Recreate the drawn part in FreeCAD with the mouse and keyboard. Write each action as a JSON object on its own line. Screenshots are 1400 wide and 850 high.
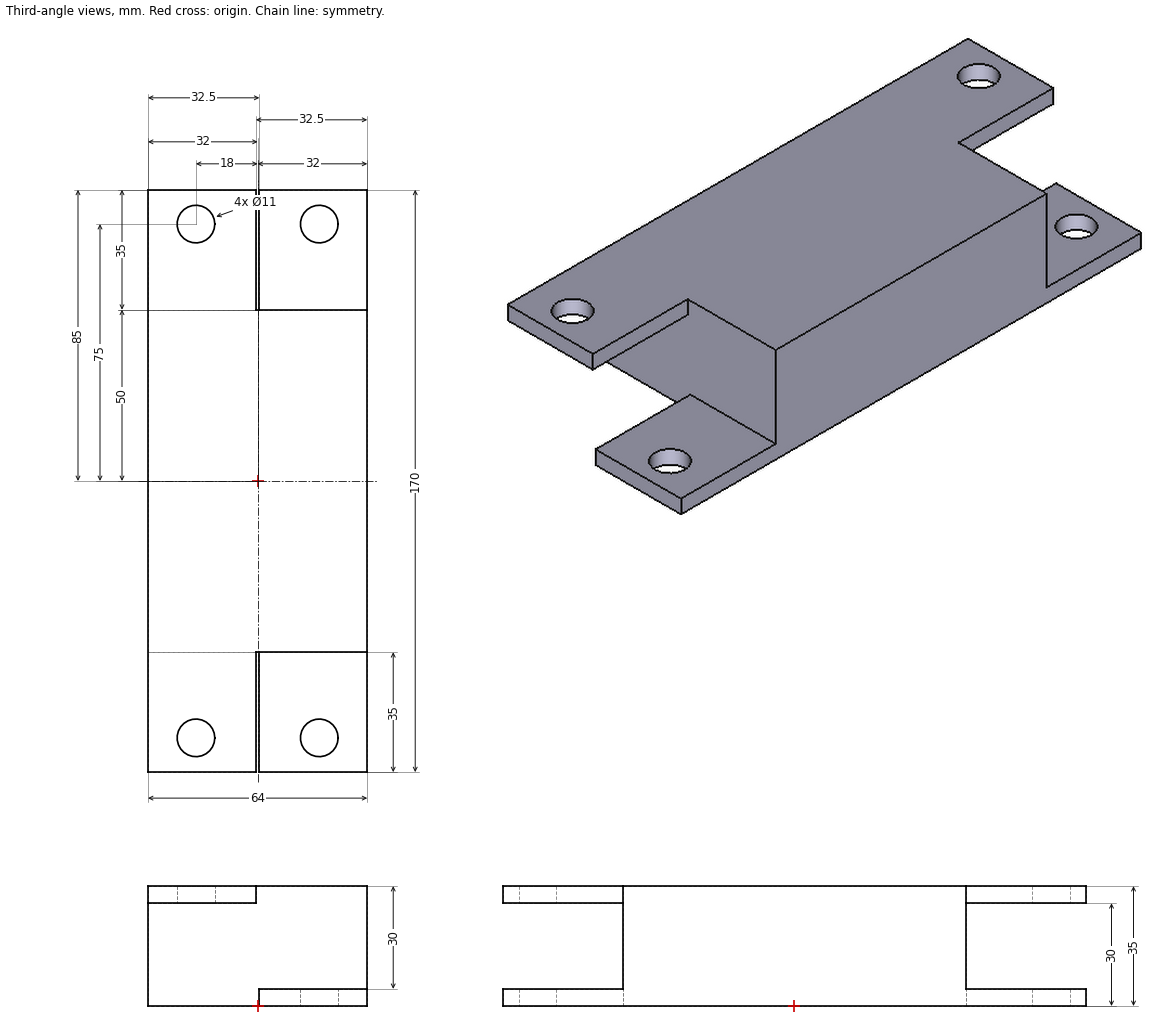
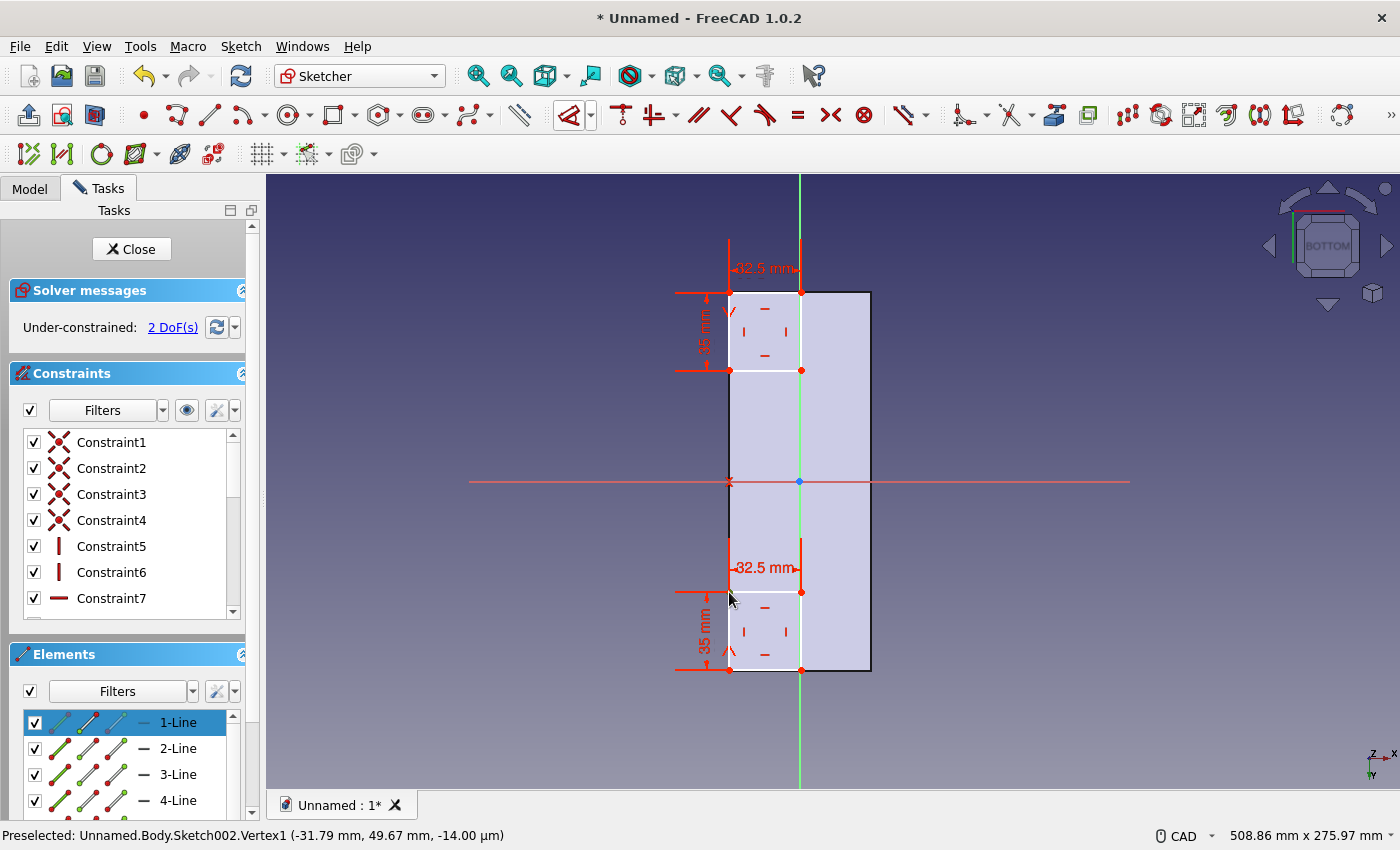
{"action": "left_click", "coordinate": [590, 116]}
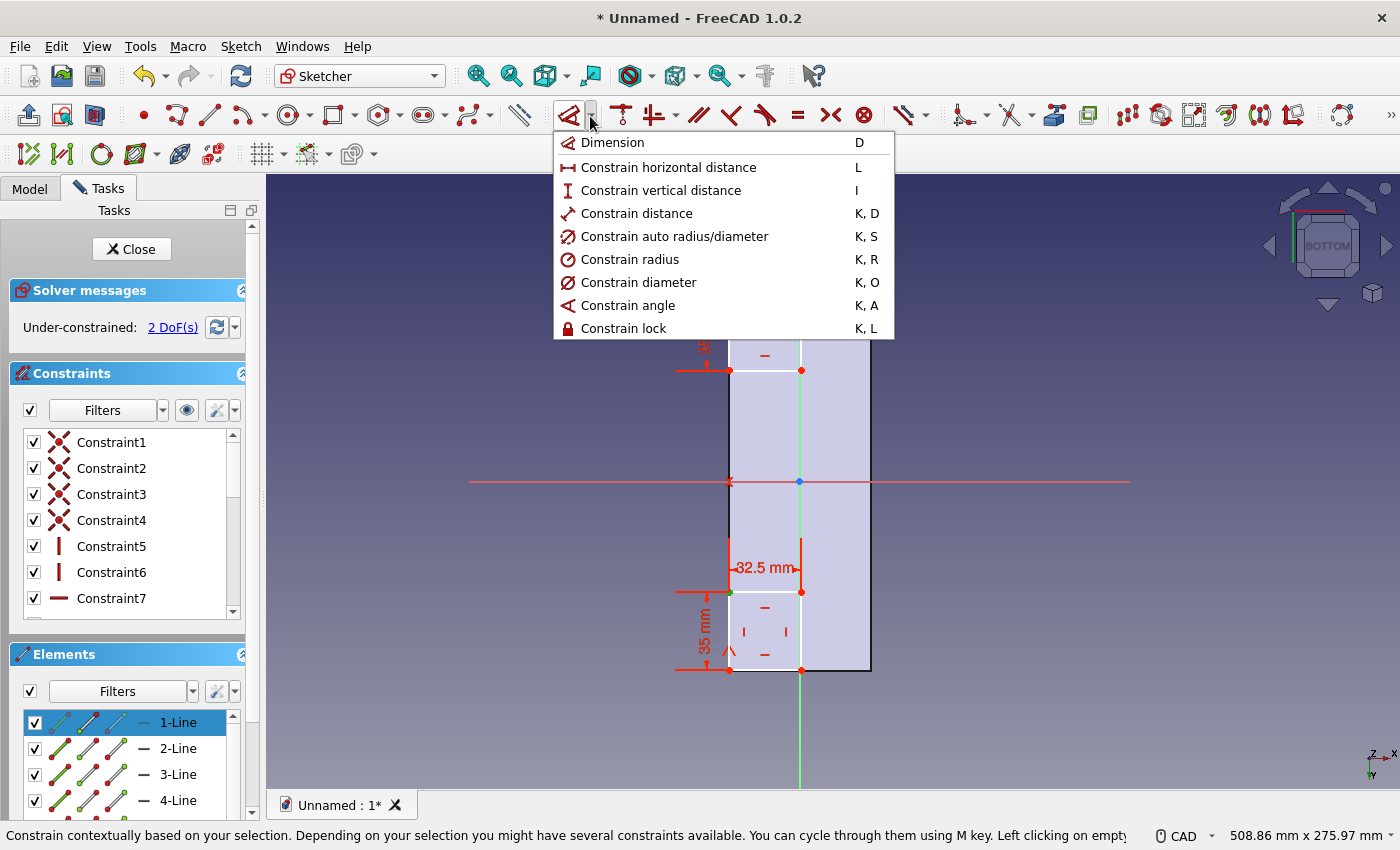
{"action": "left_click", "coordinate": [724, 168]}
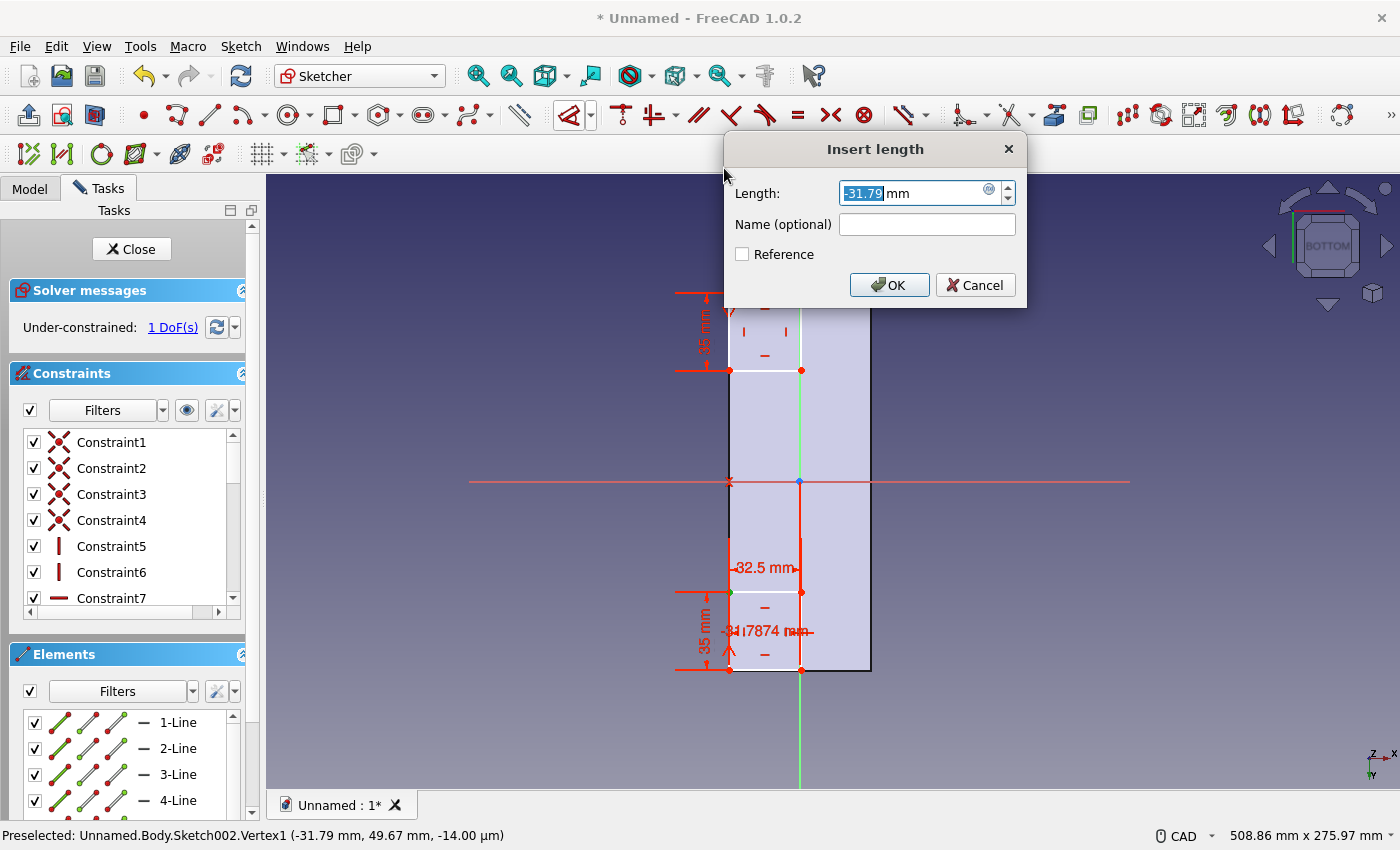
{"action": "type", "text": "-32"}
{"action": "key", "text": "Return"}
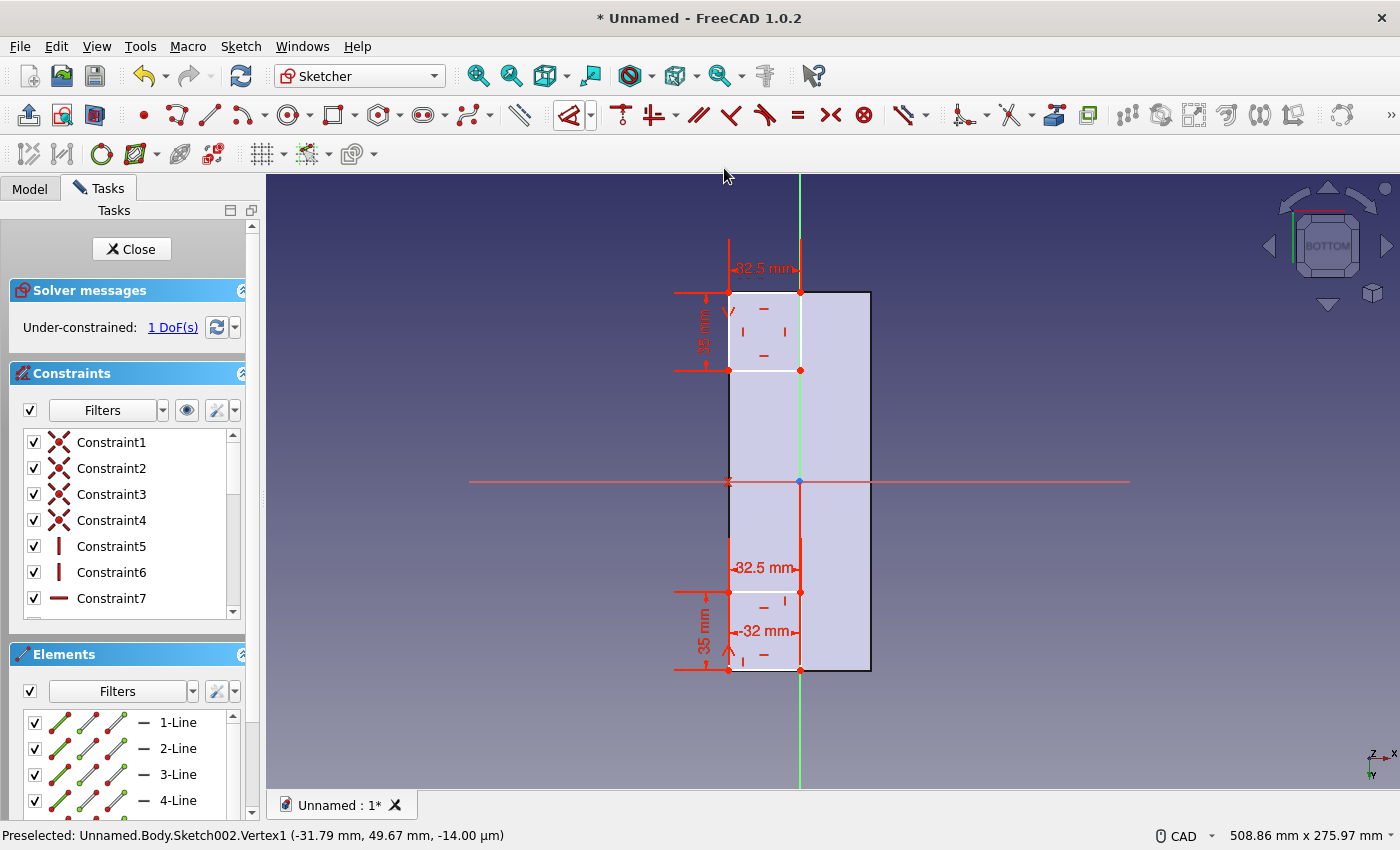
{"action": "left_click", "coordinate": [729, 592]}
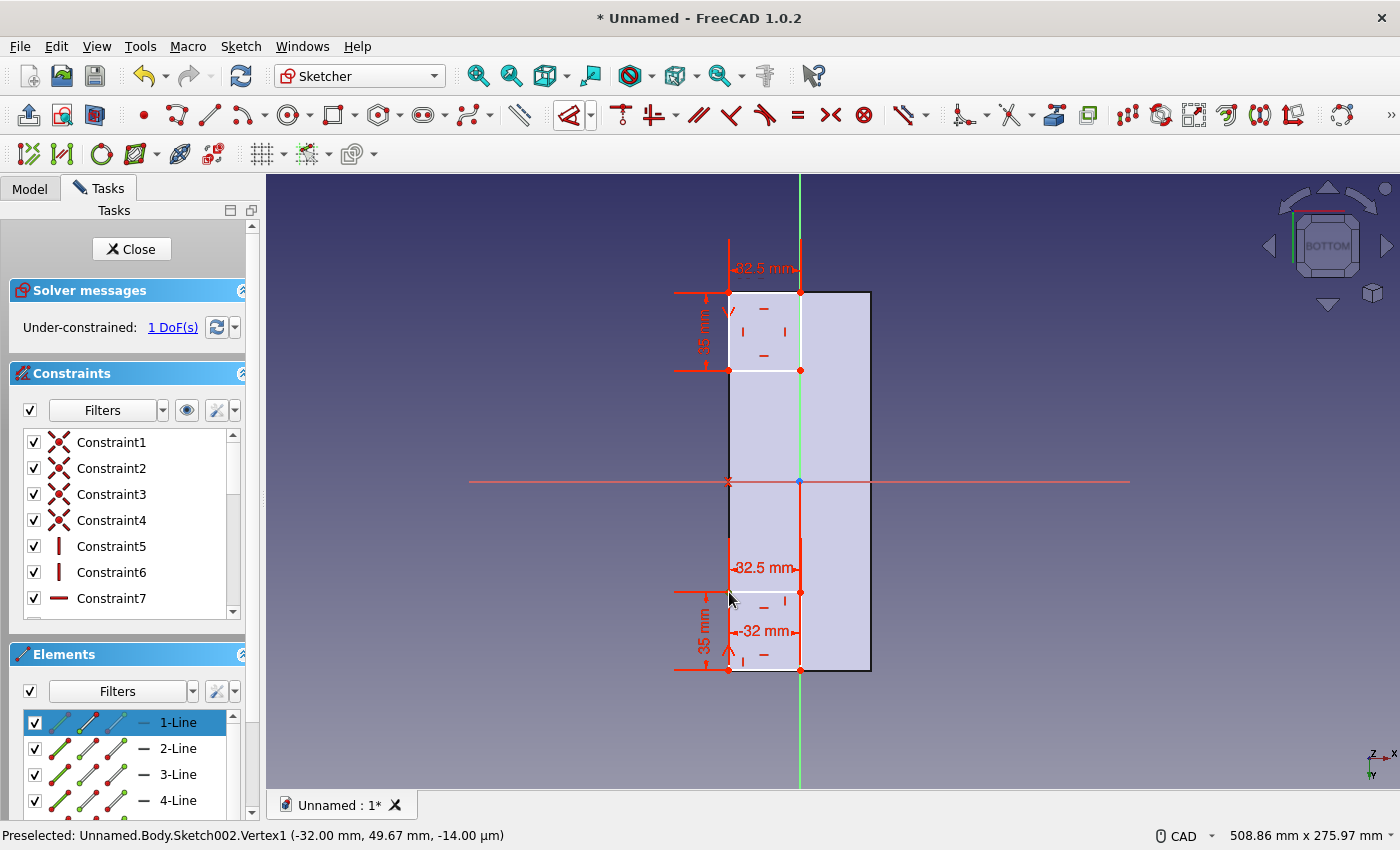
{"action": "key", "text": "i"}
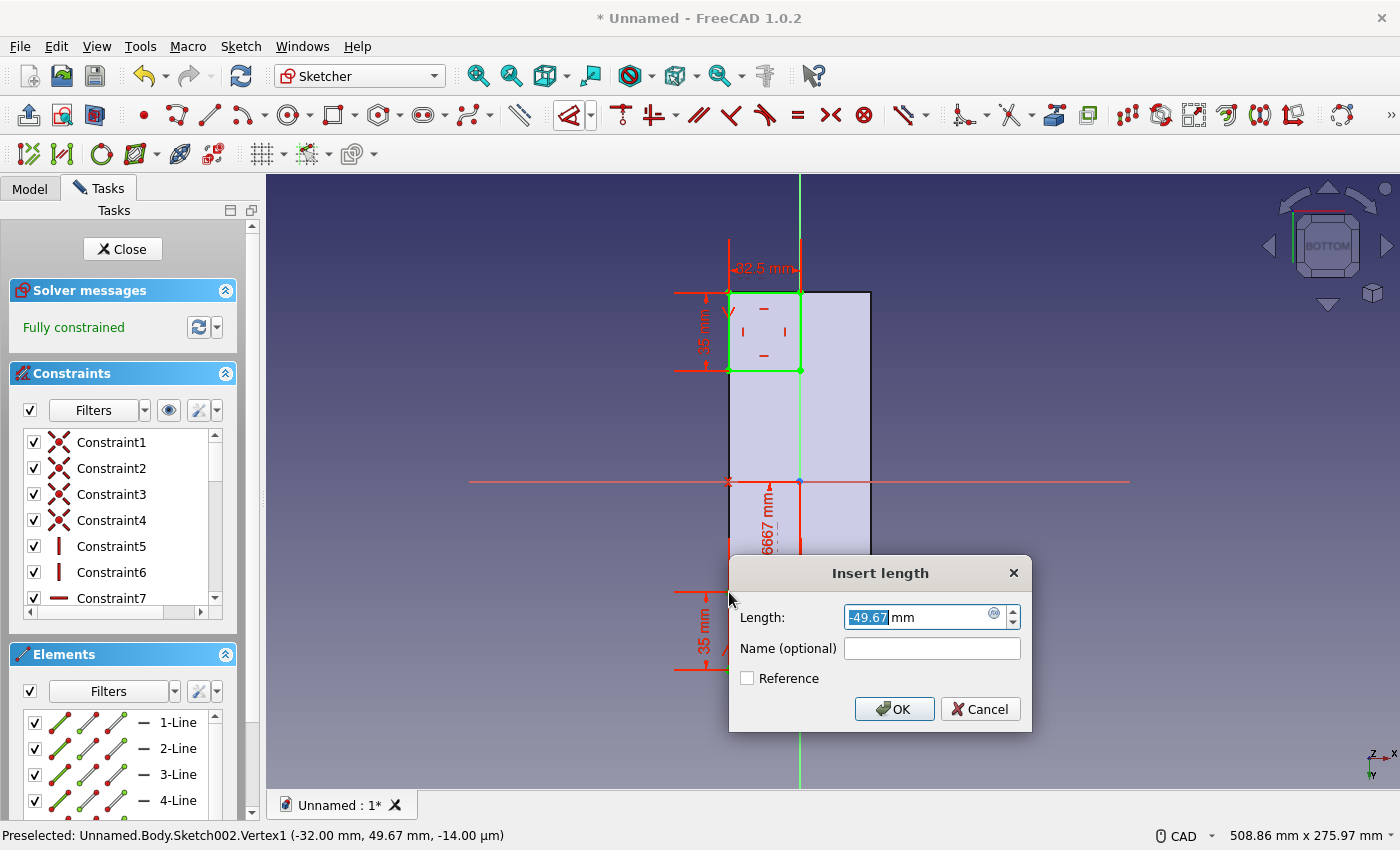
{"action": "type", "text": "-50"}
{"action": "key", "text": "Return"}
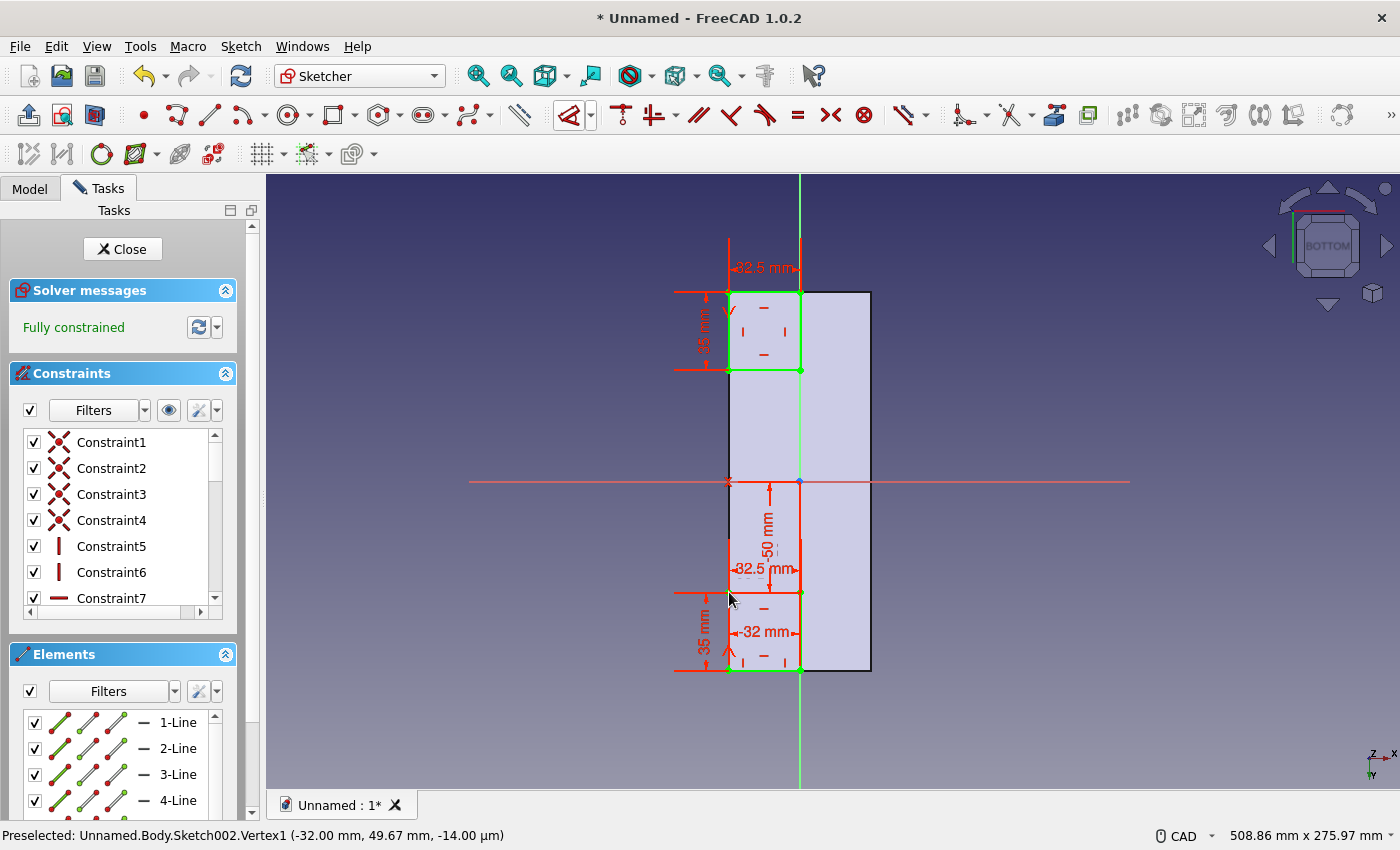
{"action": "left_click", "coordinate": [123, 249]}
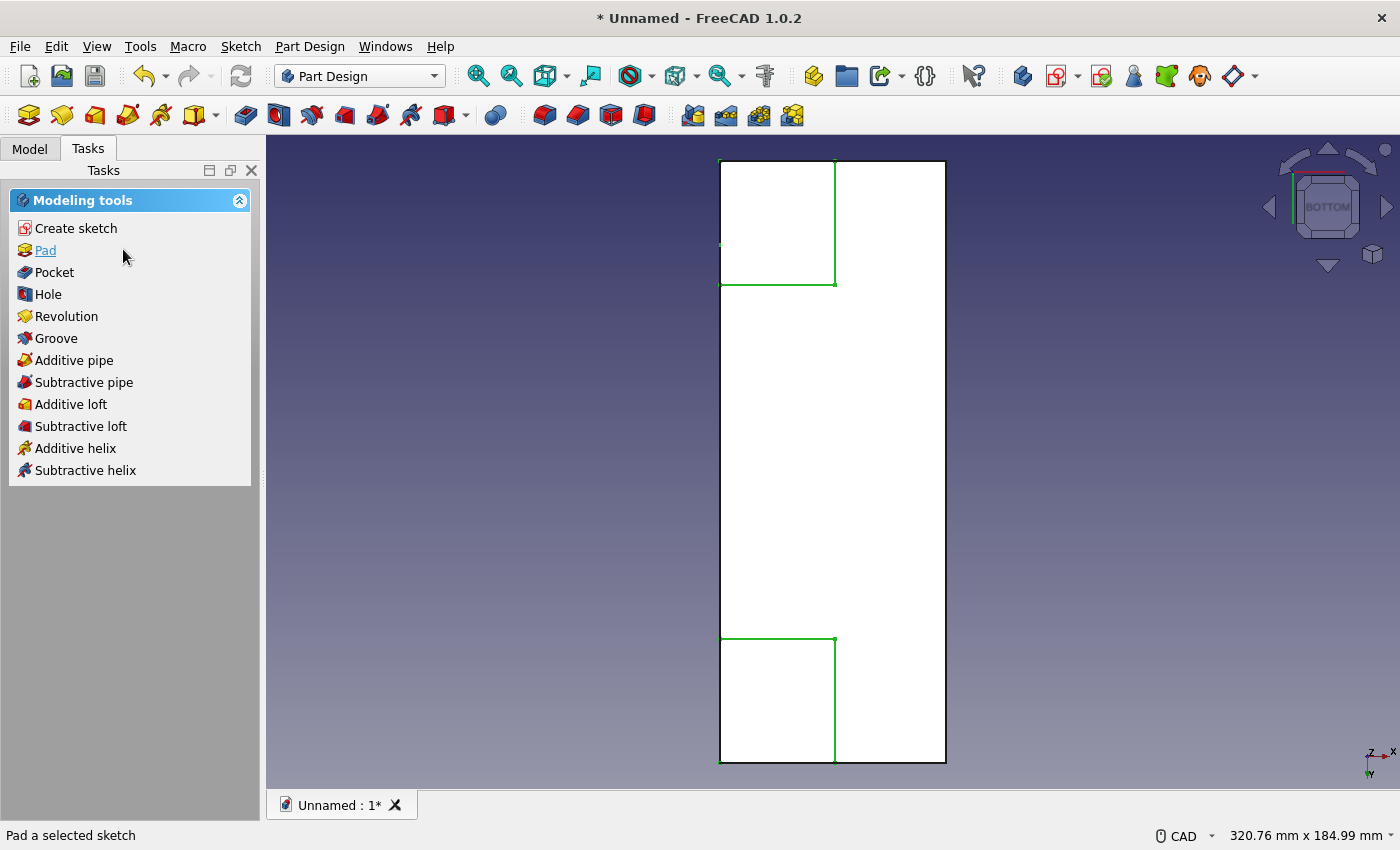
{"action": "left_click", "coordinate": [246, 116]}